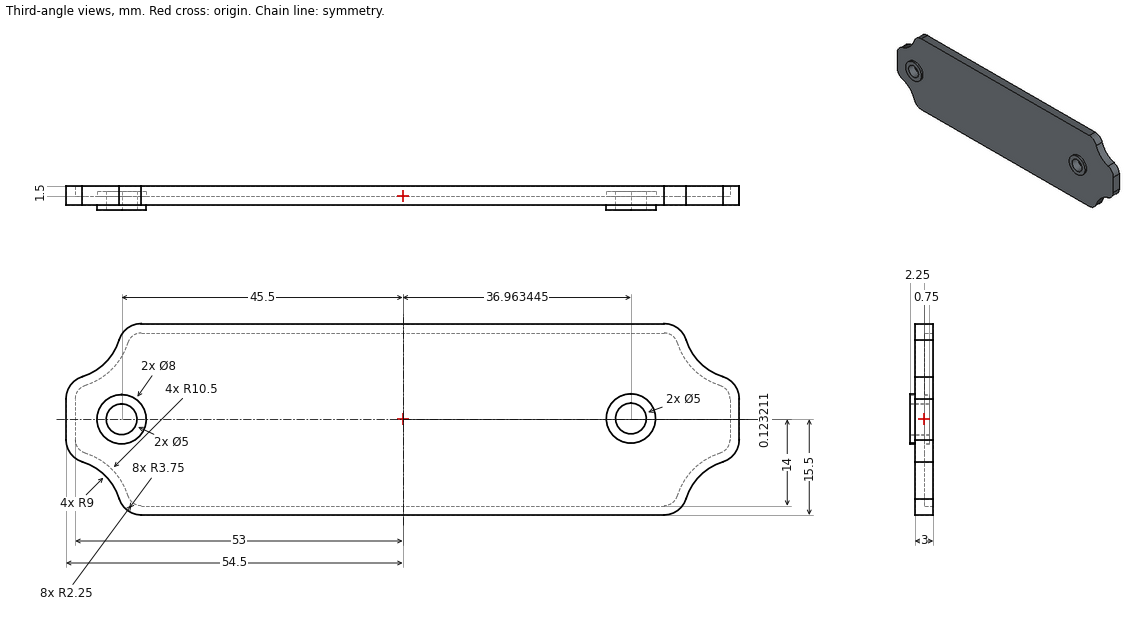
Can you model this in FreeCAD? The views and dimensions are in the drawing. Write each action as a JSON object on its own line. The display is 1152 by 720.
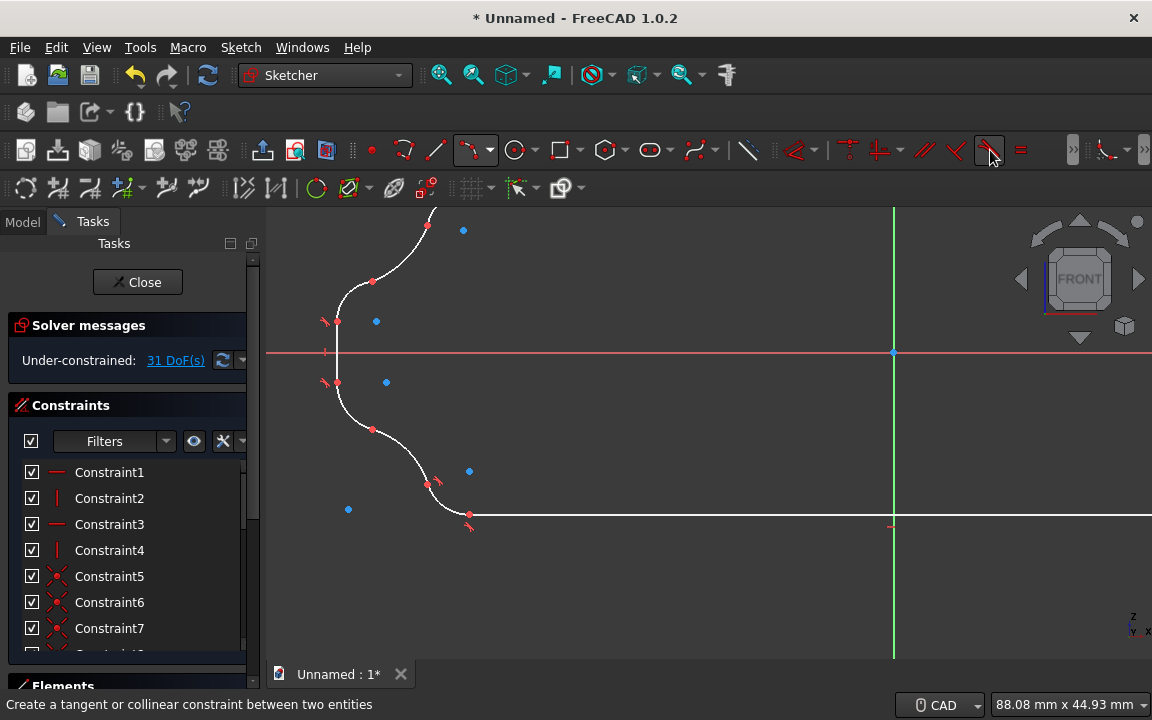
{"action": "left_click", "coordinate": [417, 462]}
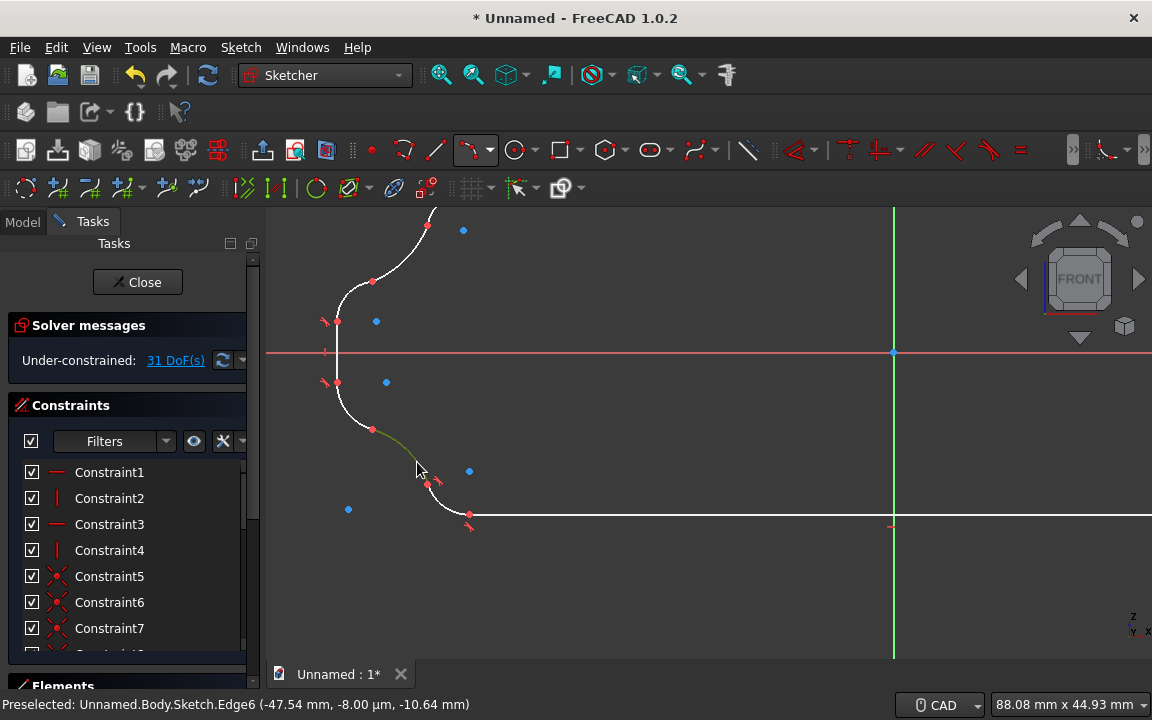
{"action": "left_click", "coordinate": [341, 401]}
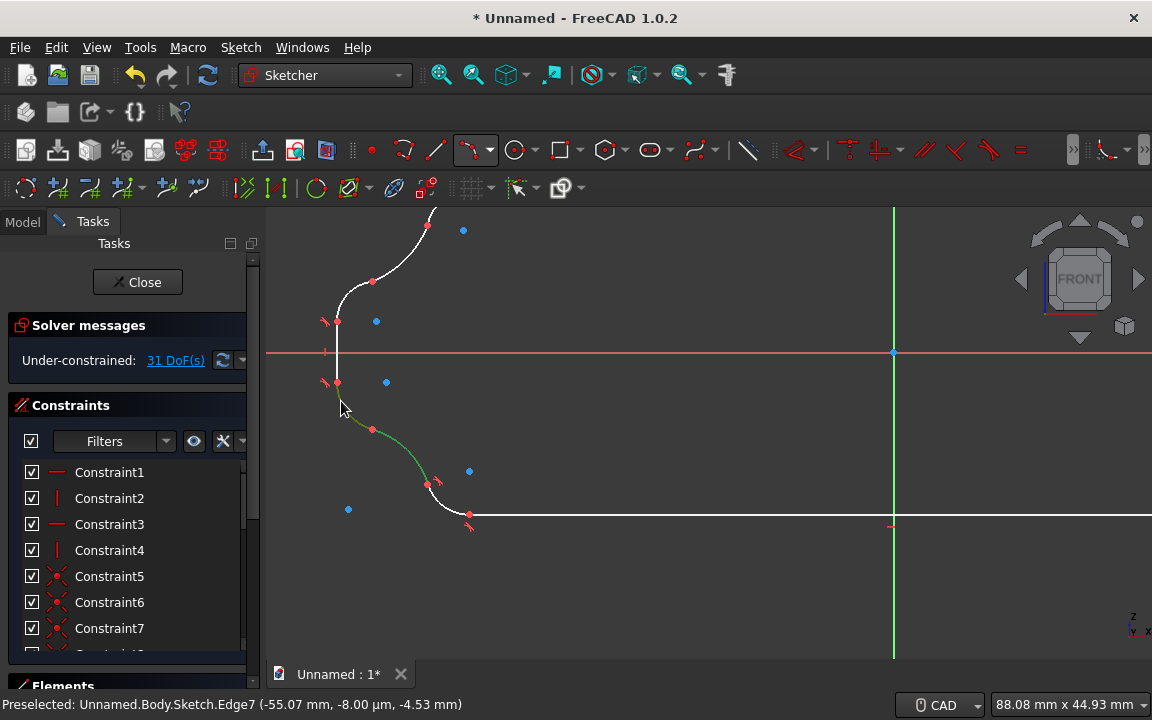
{"action": "left_click", "coordinate": [990, 150]}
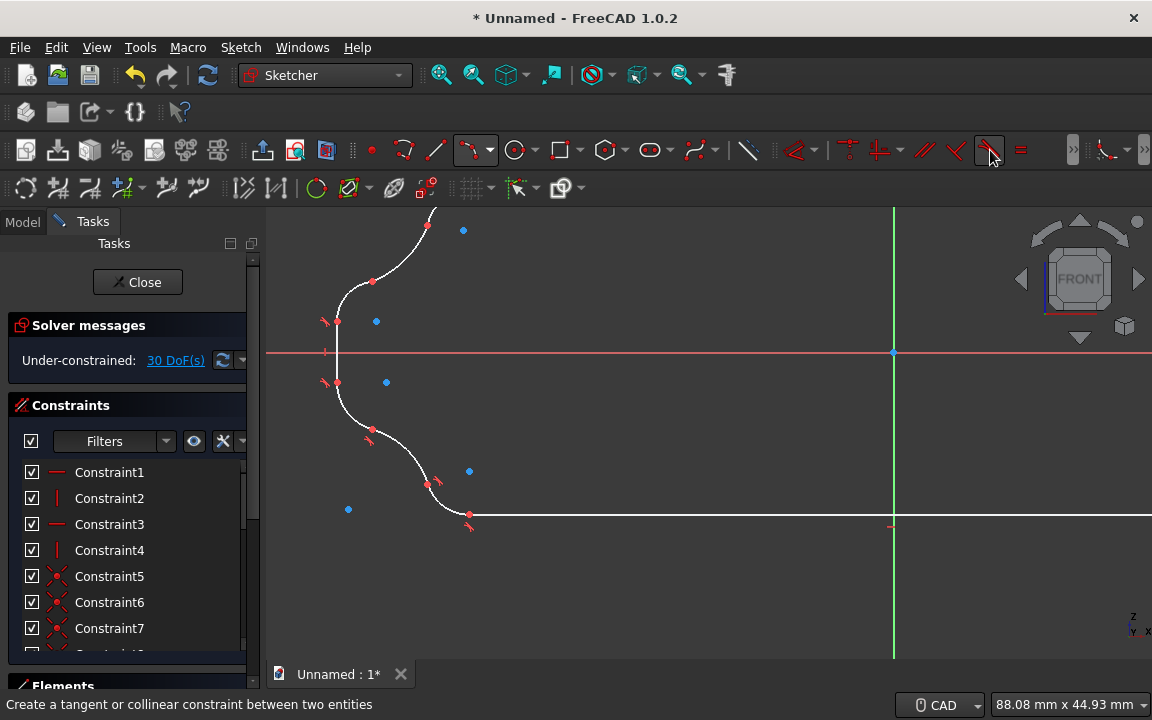
{"action": "left_click", "coordinate": [356, 287]}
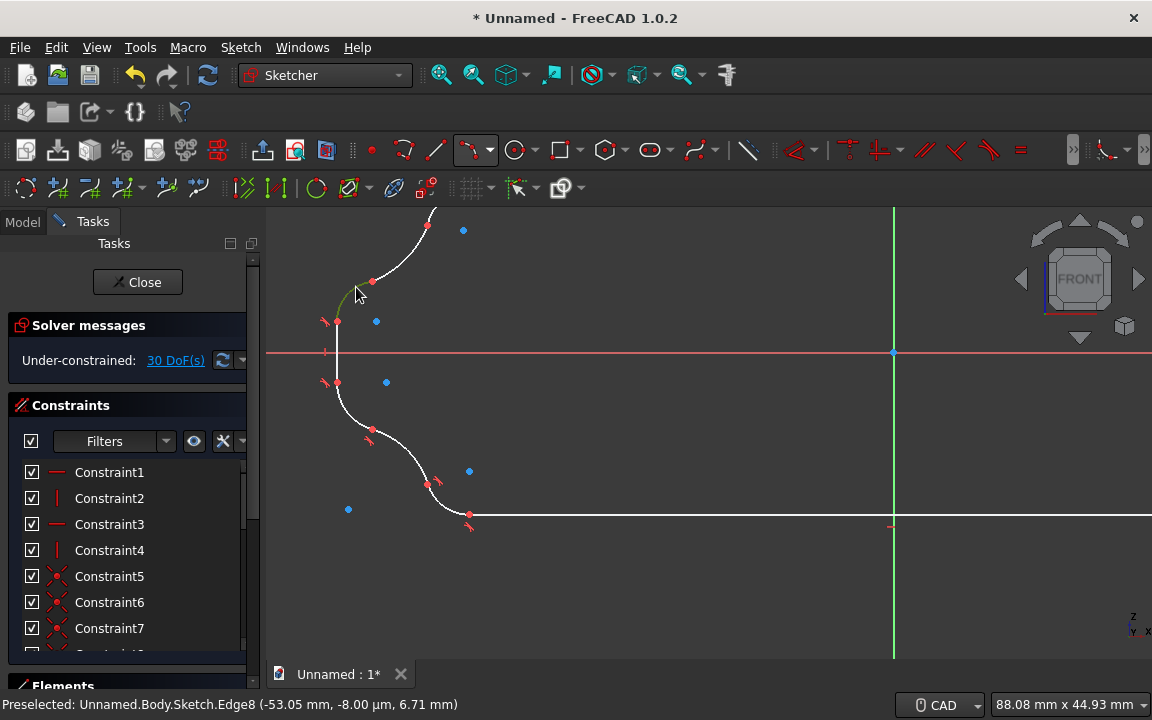
{"action": "left_click", "coordinate": [393, 270]}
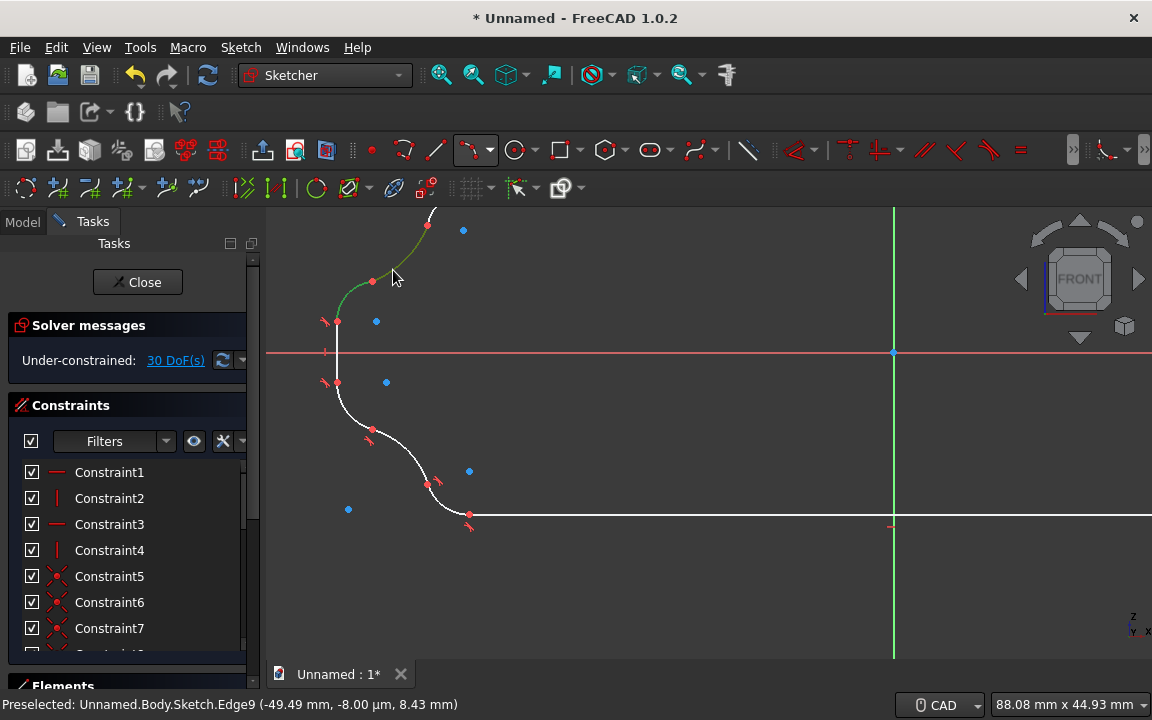
{"action": "left_click", "coordinate": [990, 150]}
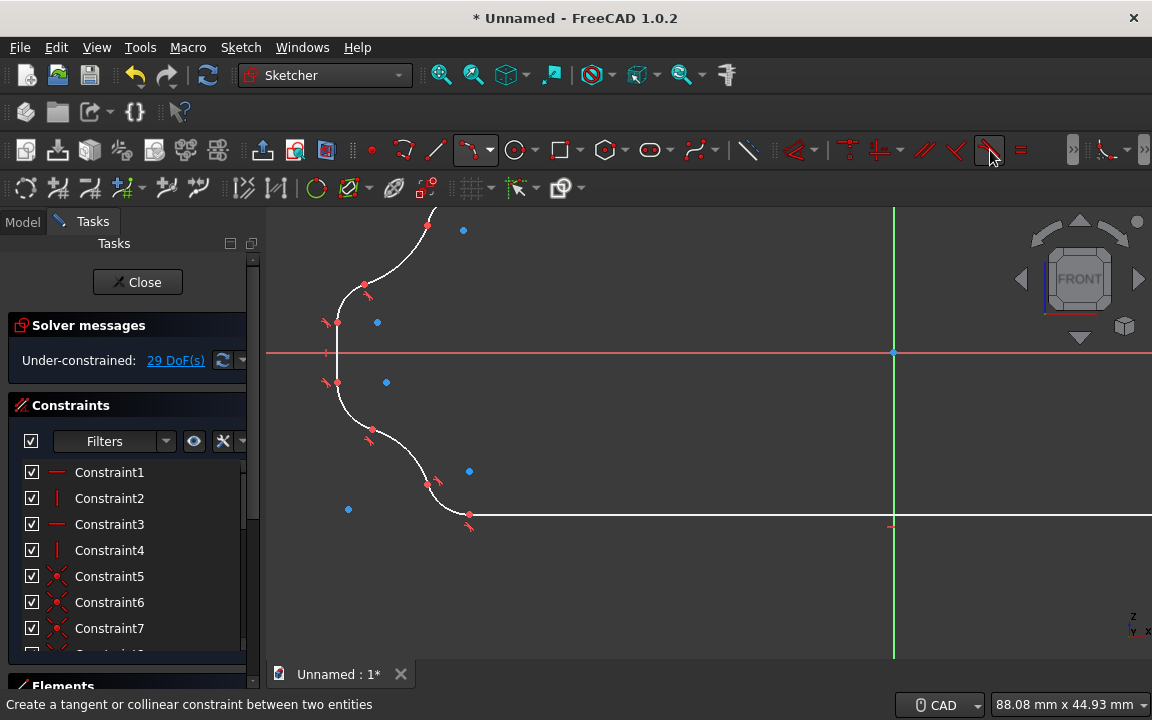
{"action": "left_click", "coordinate": [389, 273]}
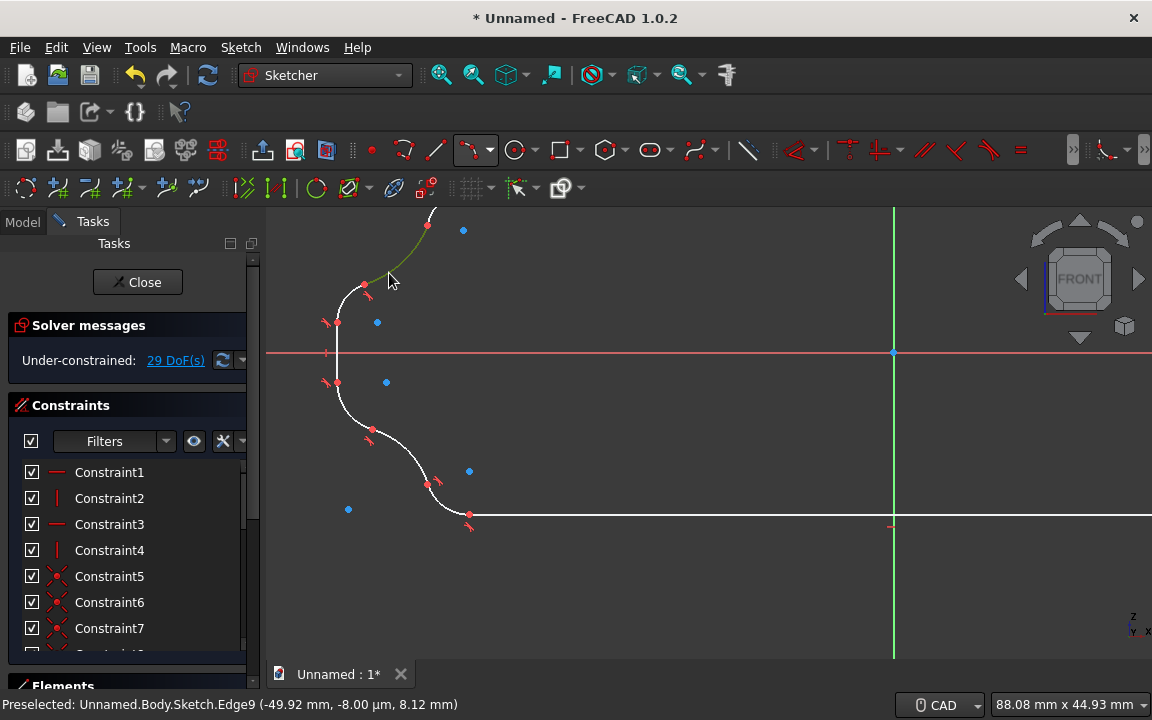
{"action": "scroll", "coordinate": [434, 499], "scroll_direction": "down", "scroll_amount": 4}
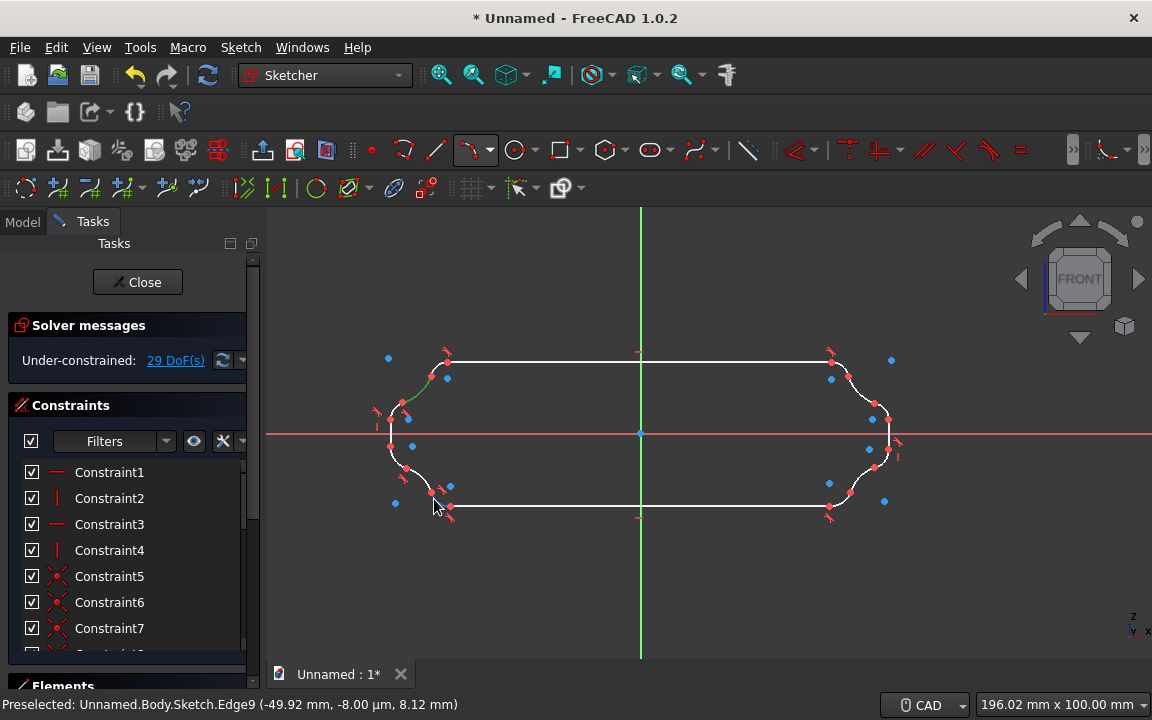
{"action": "scroll", "coordinate": [441, 364], "scroll_direction": "up", "scroll_amount": 4}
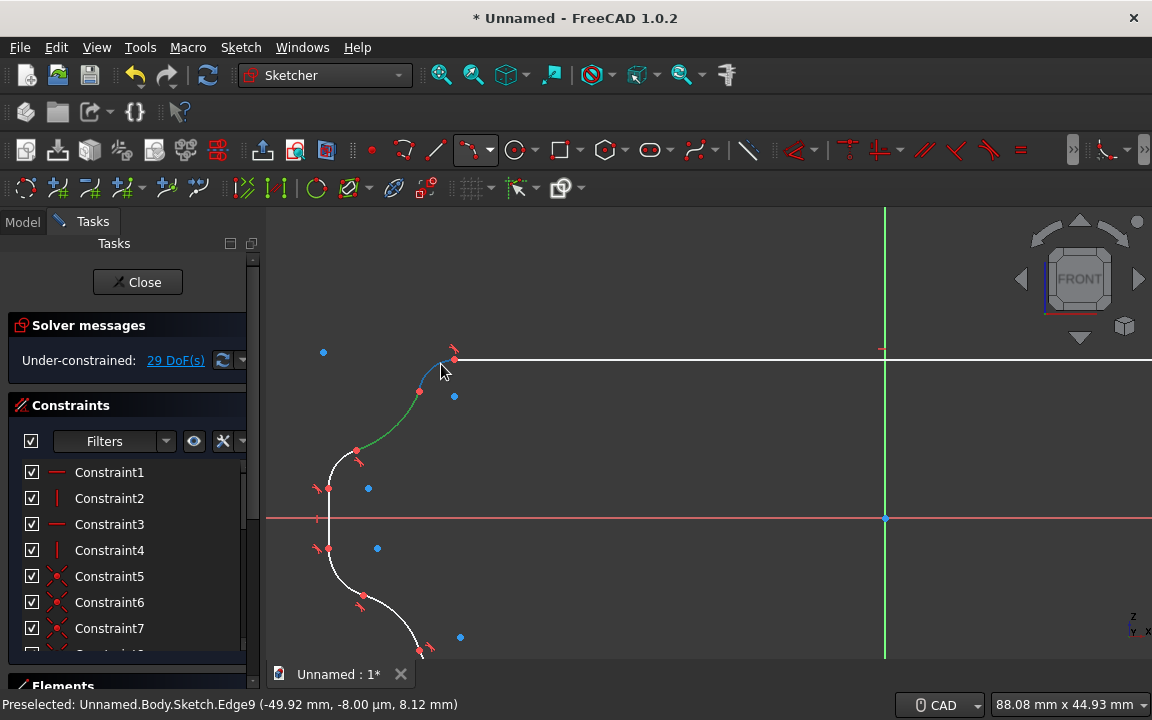
{"action": "left_click", "coordinate": [440, 363]}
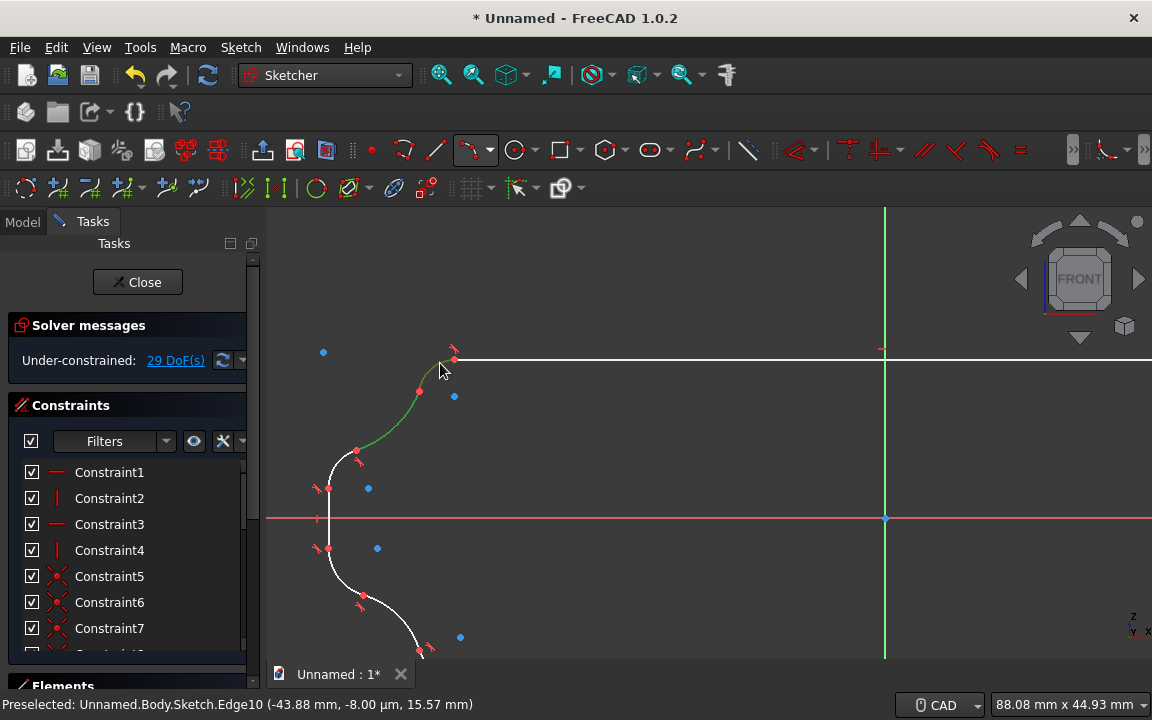
{"action": "left_click", "coordinate": [990, 150]}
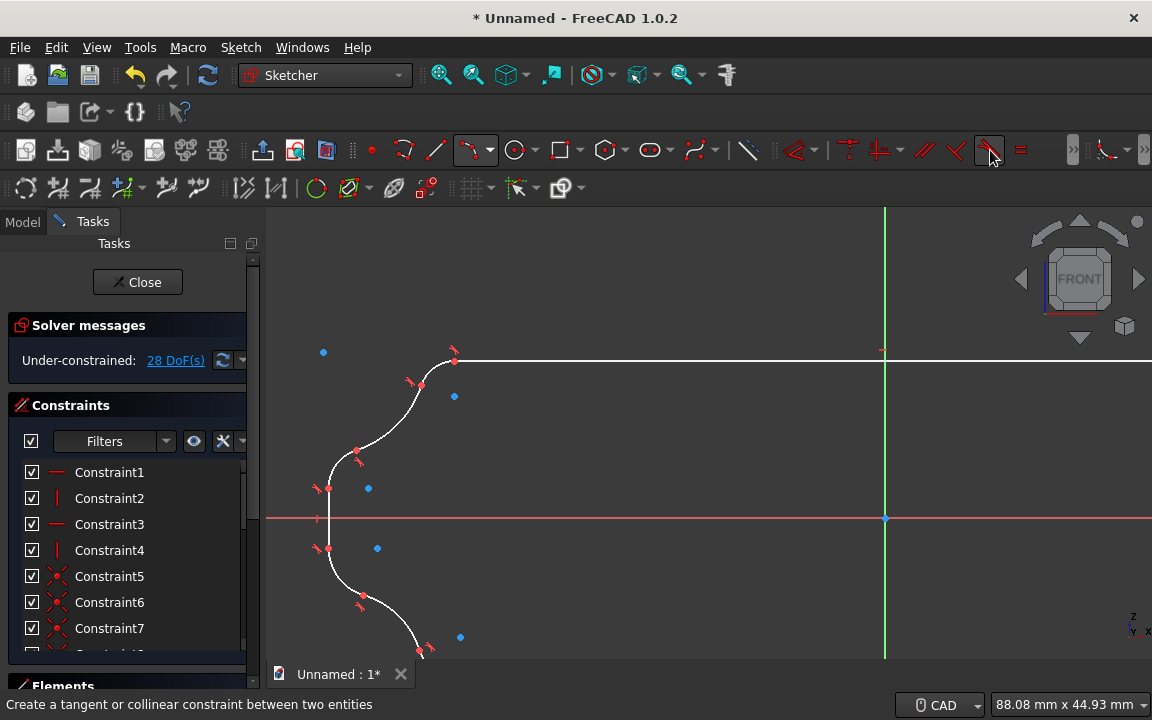
{"action": "scroll", "coordinate": [441, 363], "scroll_direction": "down", "scroll_amount": 4}